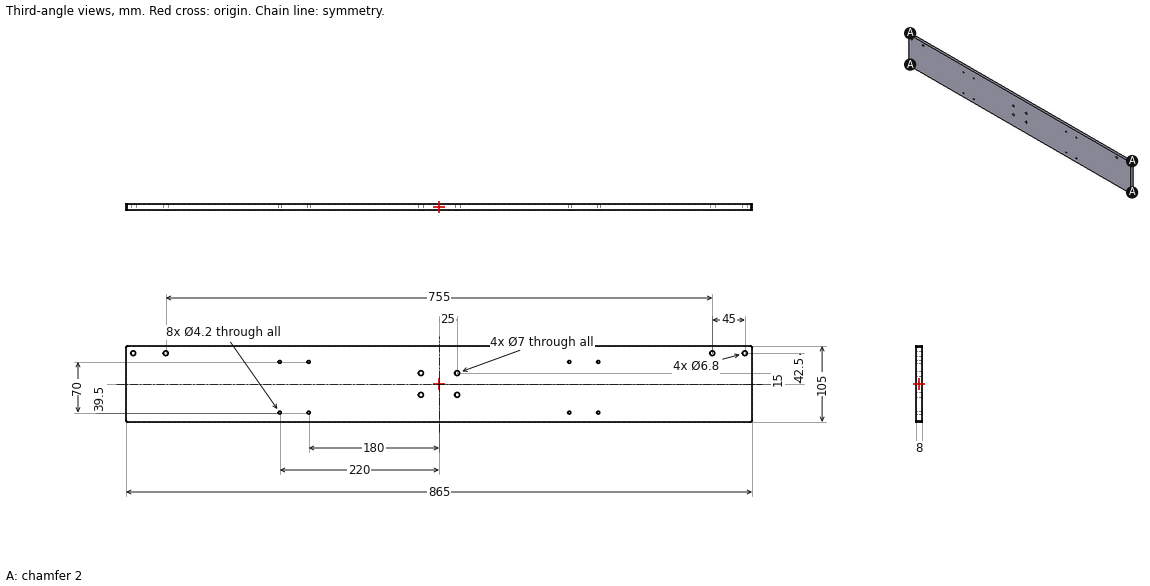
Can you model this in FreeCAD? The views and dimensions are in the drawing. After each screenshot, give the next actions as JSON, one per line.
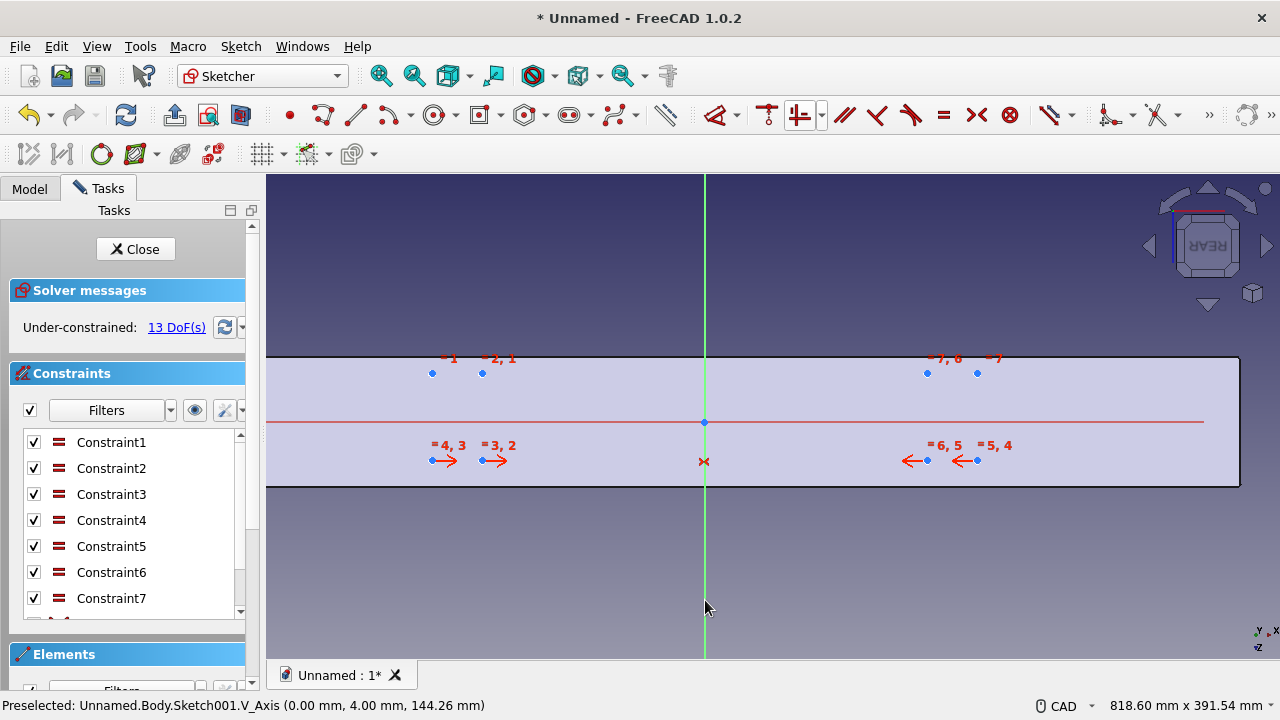
{"action": "left_click", "coordinate": [482, 374]}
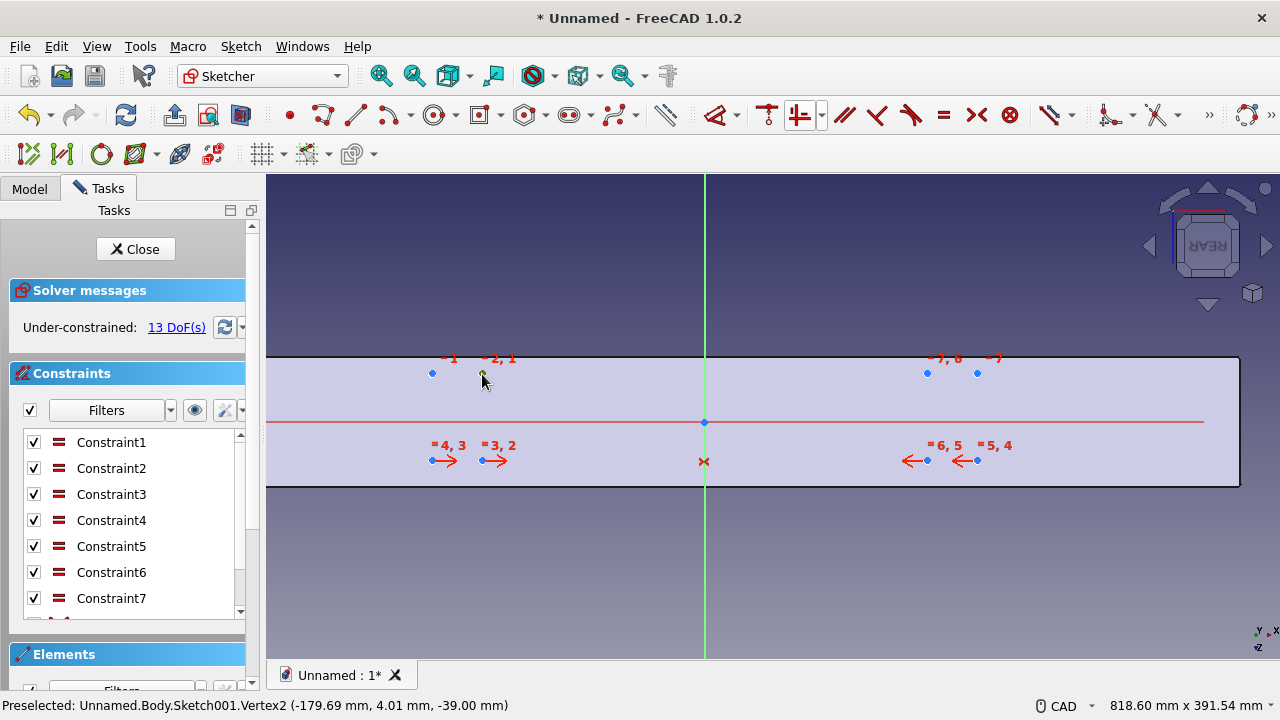
{"action": "left_click", "coordinate": [927, 374]}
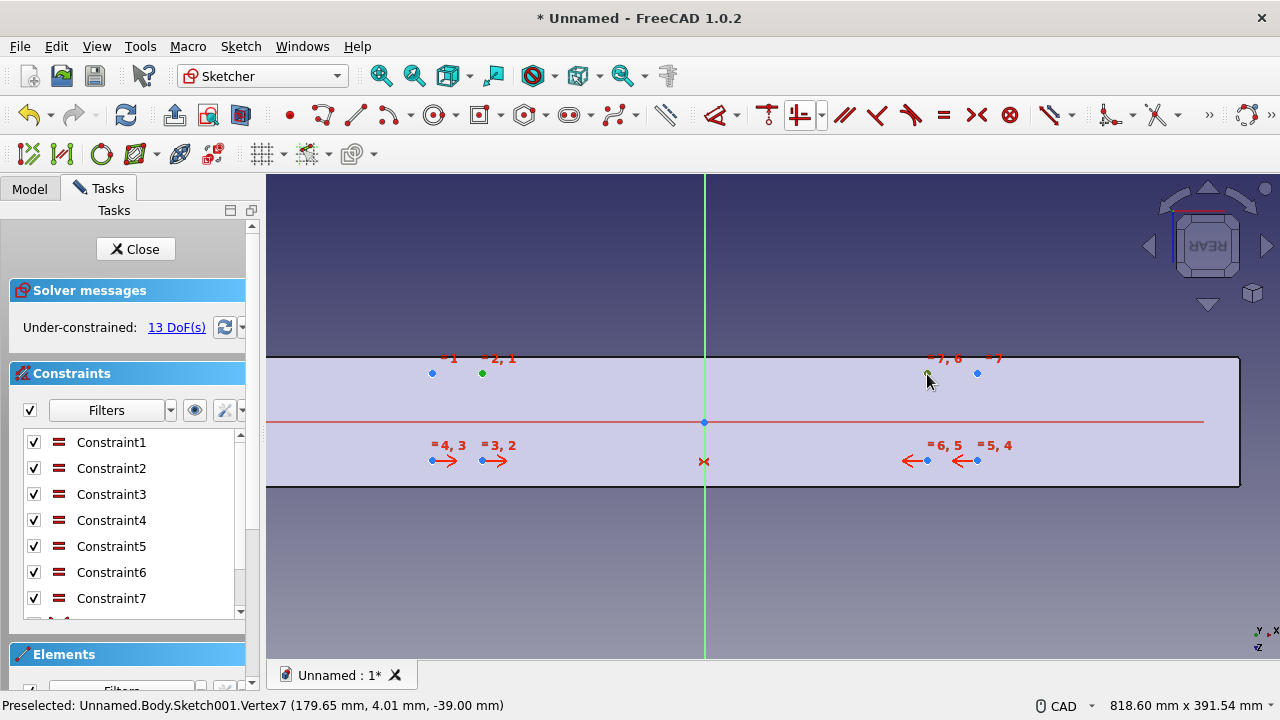
{"action": "left_click", "coordinate": [705, 600]}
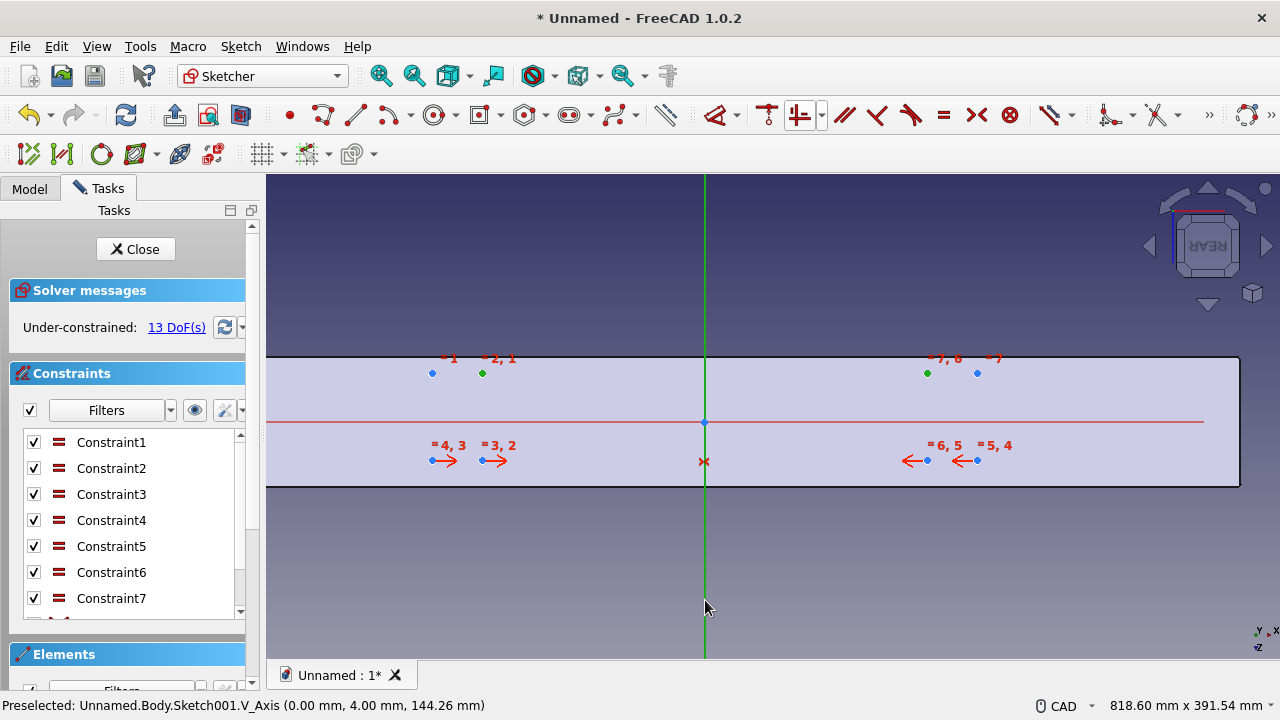
{"action": "key", "text": "s"}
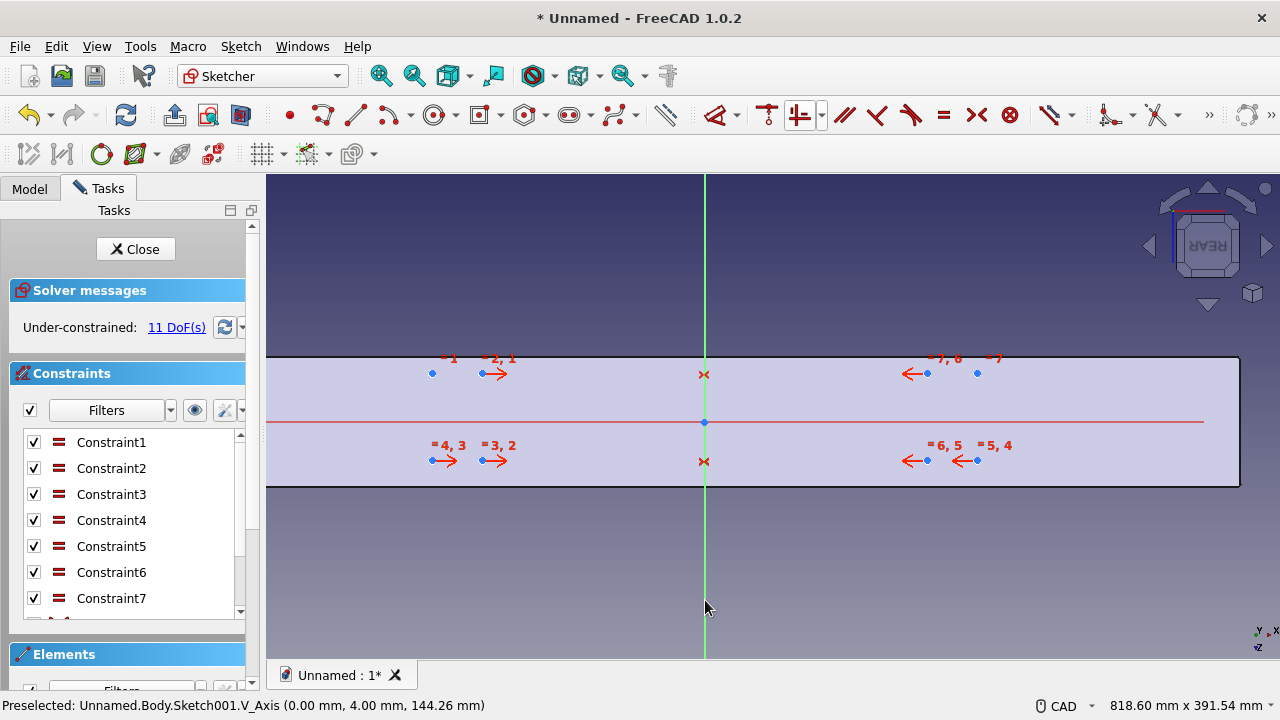
{"action": "left_click", "coordinate": [432, 374]}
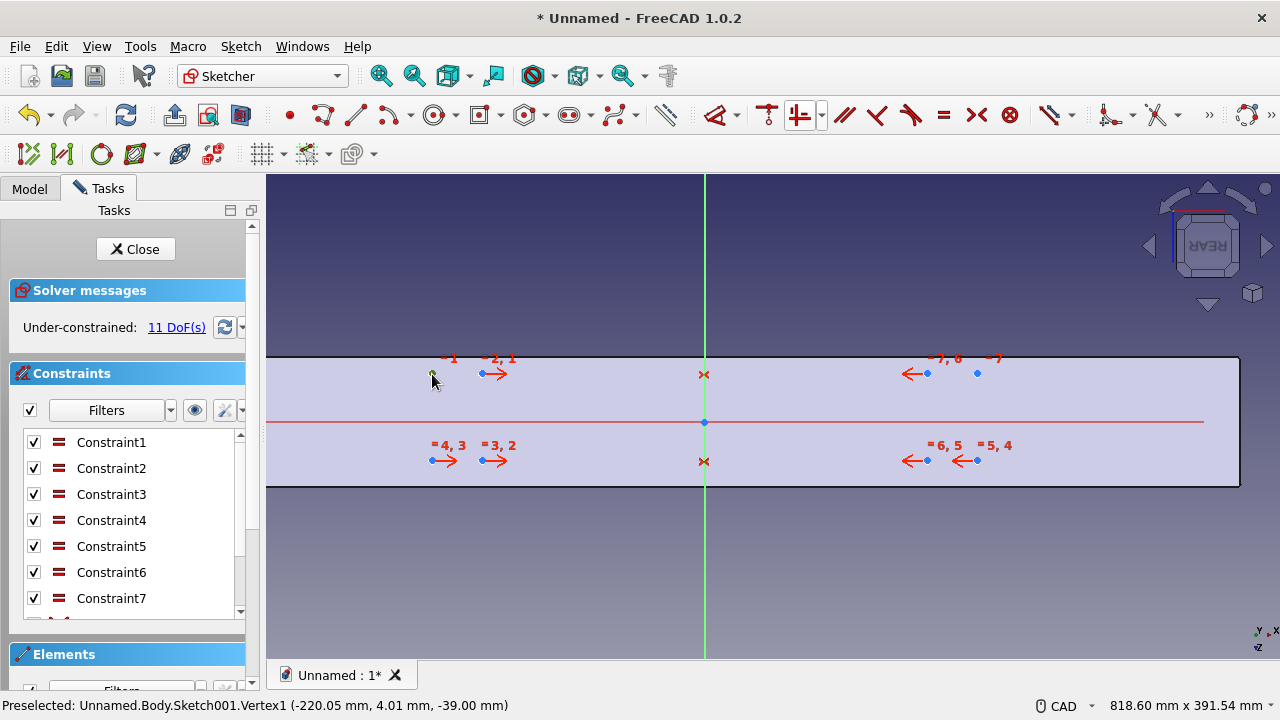
{"action": "left_click", "coordinate": [977, 374]}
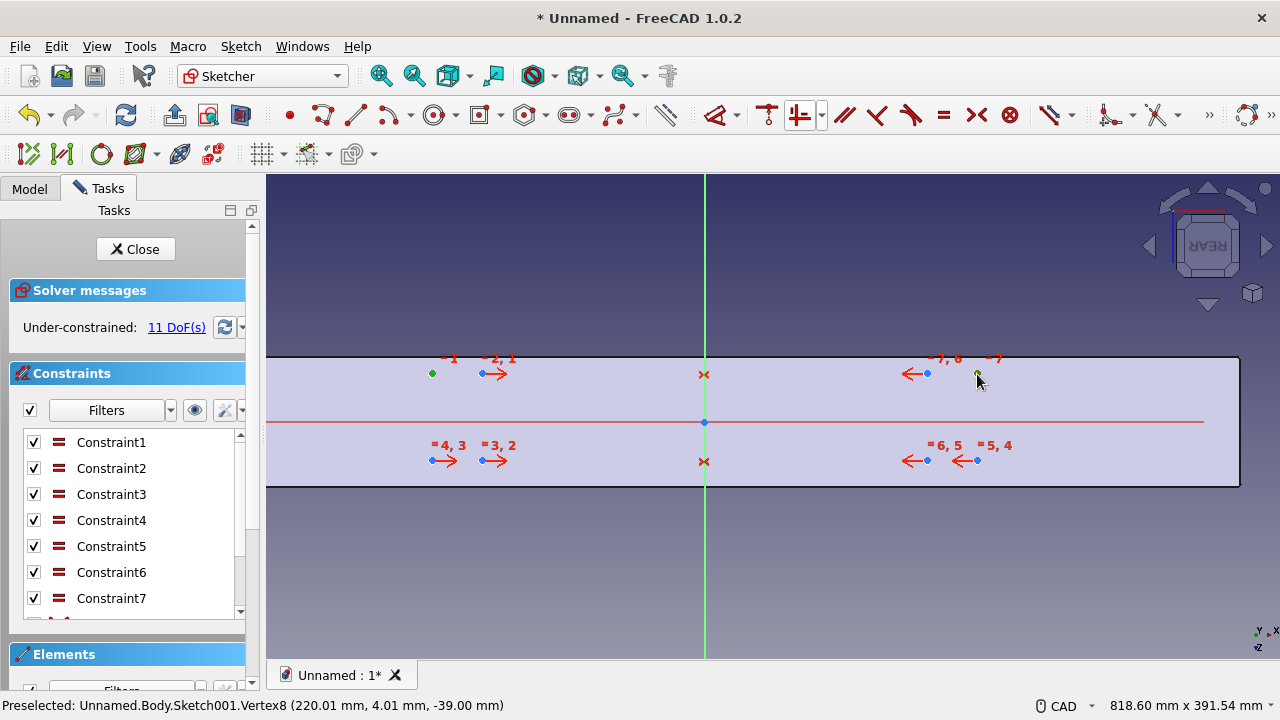
{"action": "left_click", "coordinate": [705, 600]}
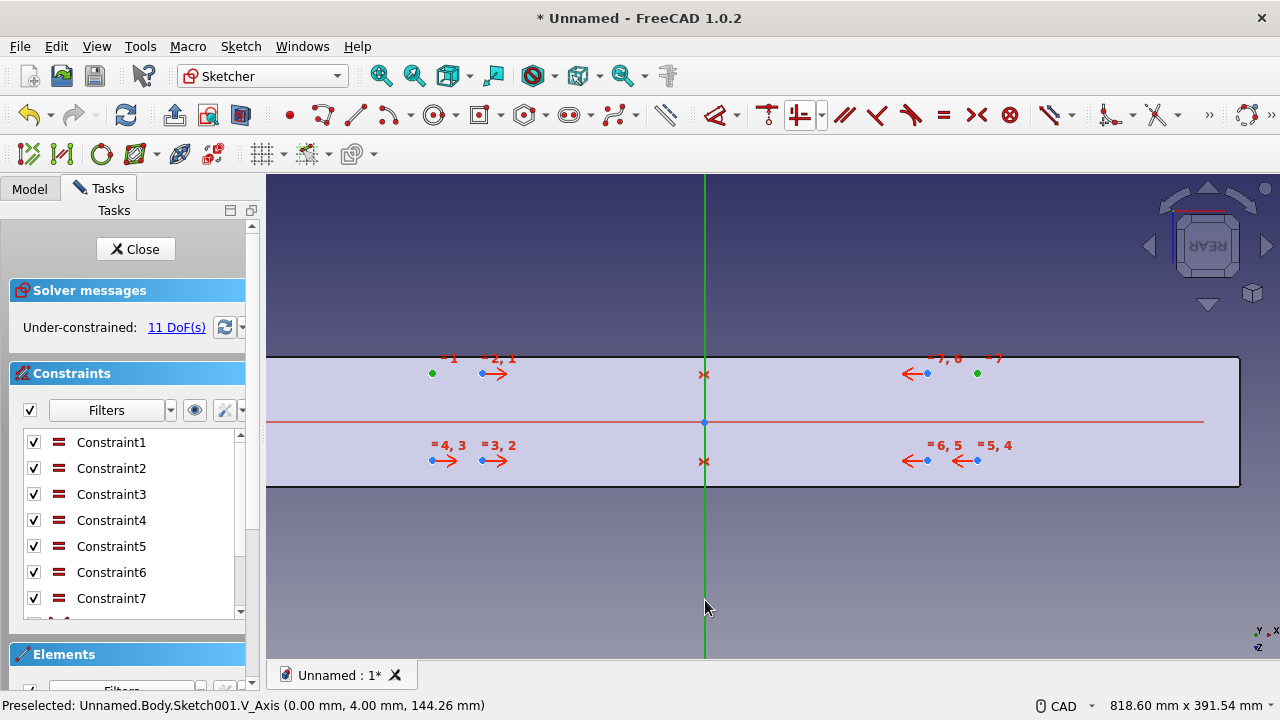
{"action": "left_click", "coordinate": [977, 116]}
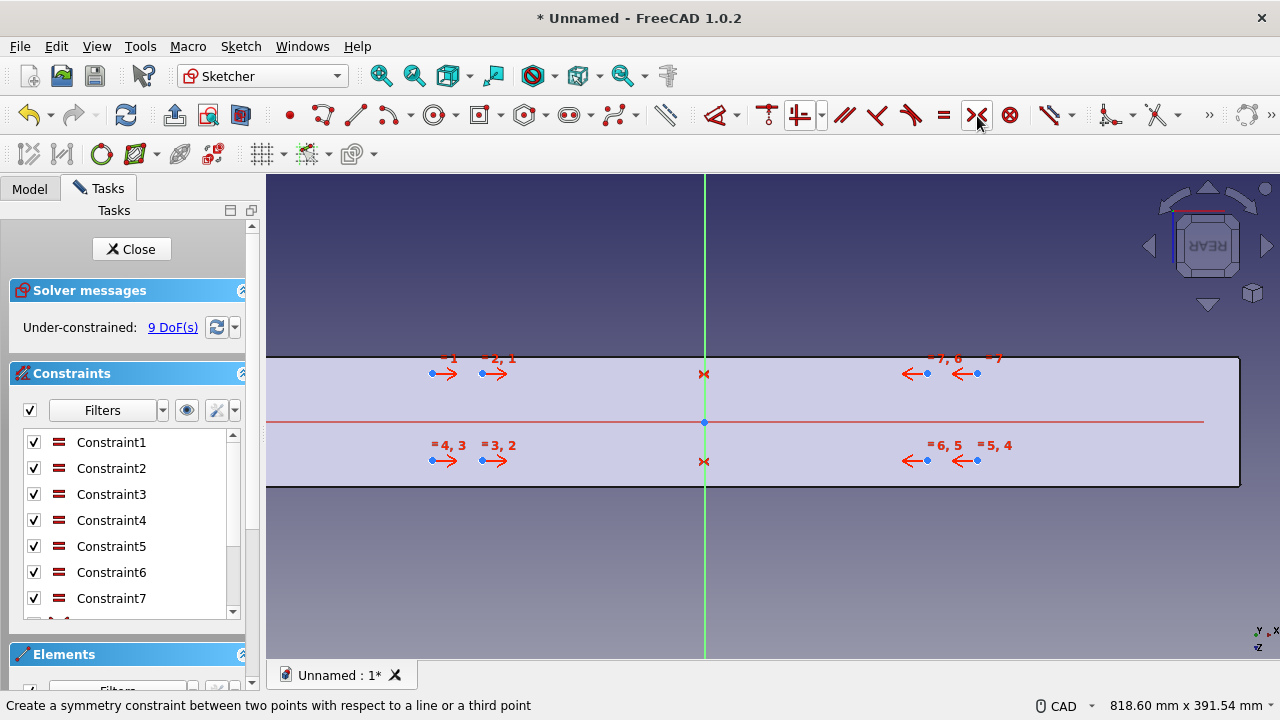
{"action": "key", "text": "d"}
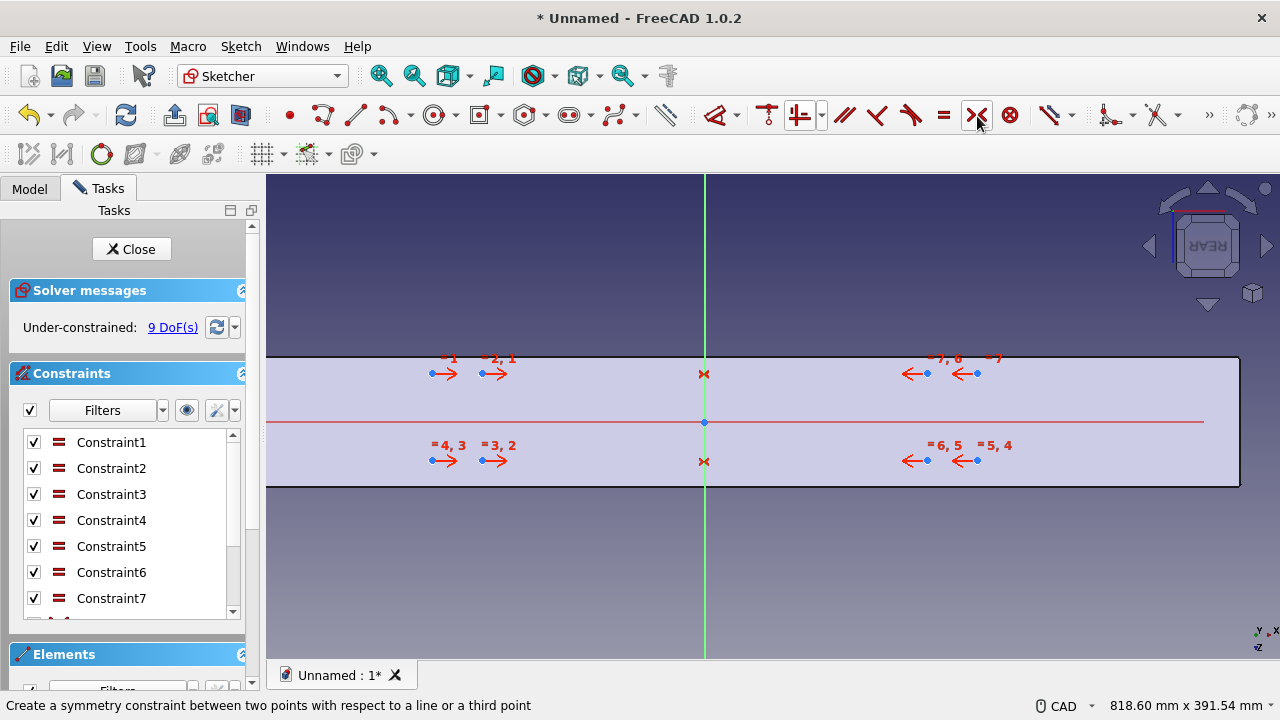
{"action": "scroll", "coordinate": [429, 374], "scroll_direction": "up", "scroll_amount": 11}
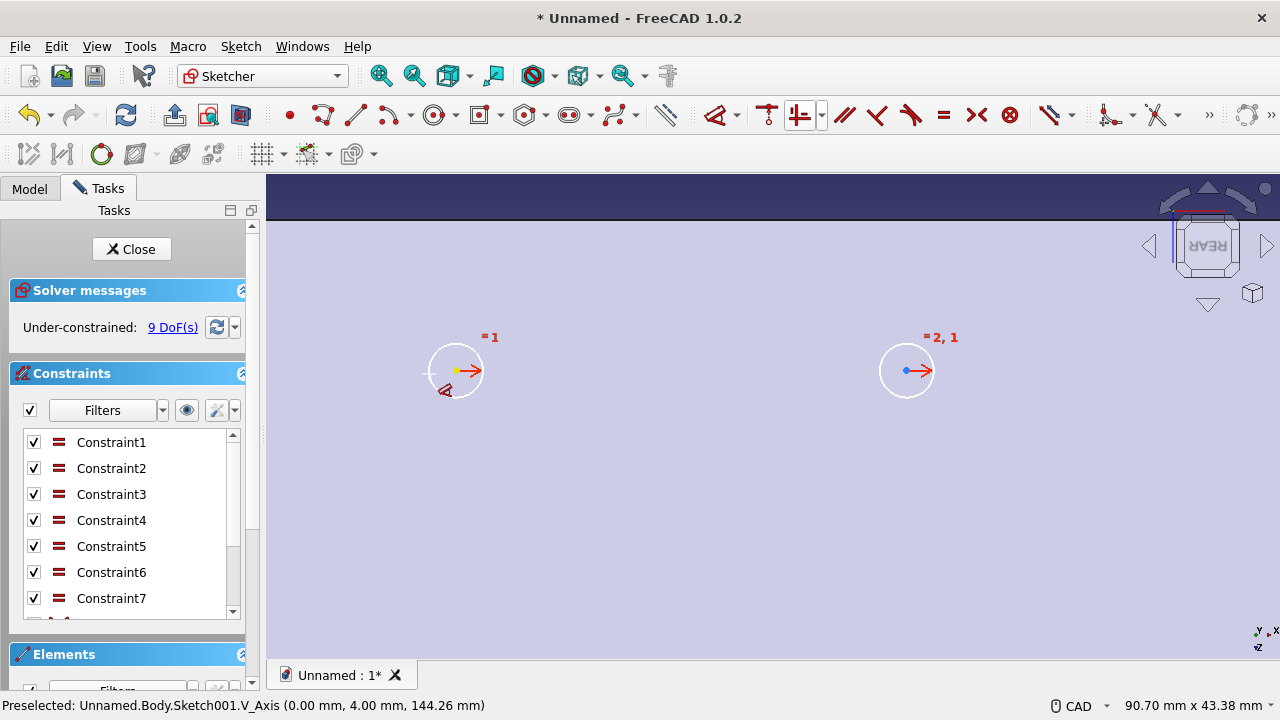
{"action": "left_click", "coordinate": [429, 370]}
{"action": "left_click", "coordinate": [397, 369]}